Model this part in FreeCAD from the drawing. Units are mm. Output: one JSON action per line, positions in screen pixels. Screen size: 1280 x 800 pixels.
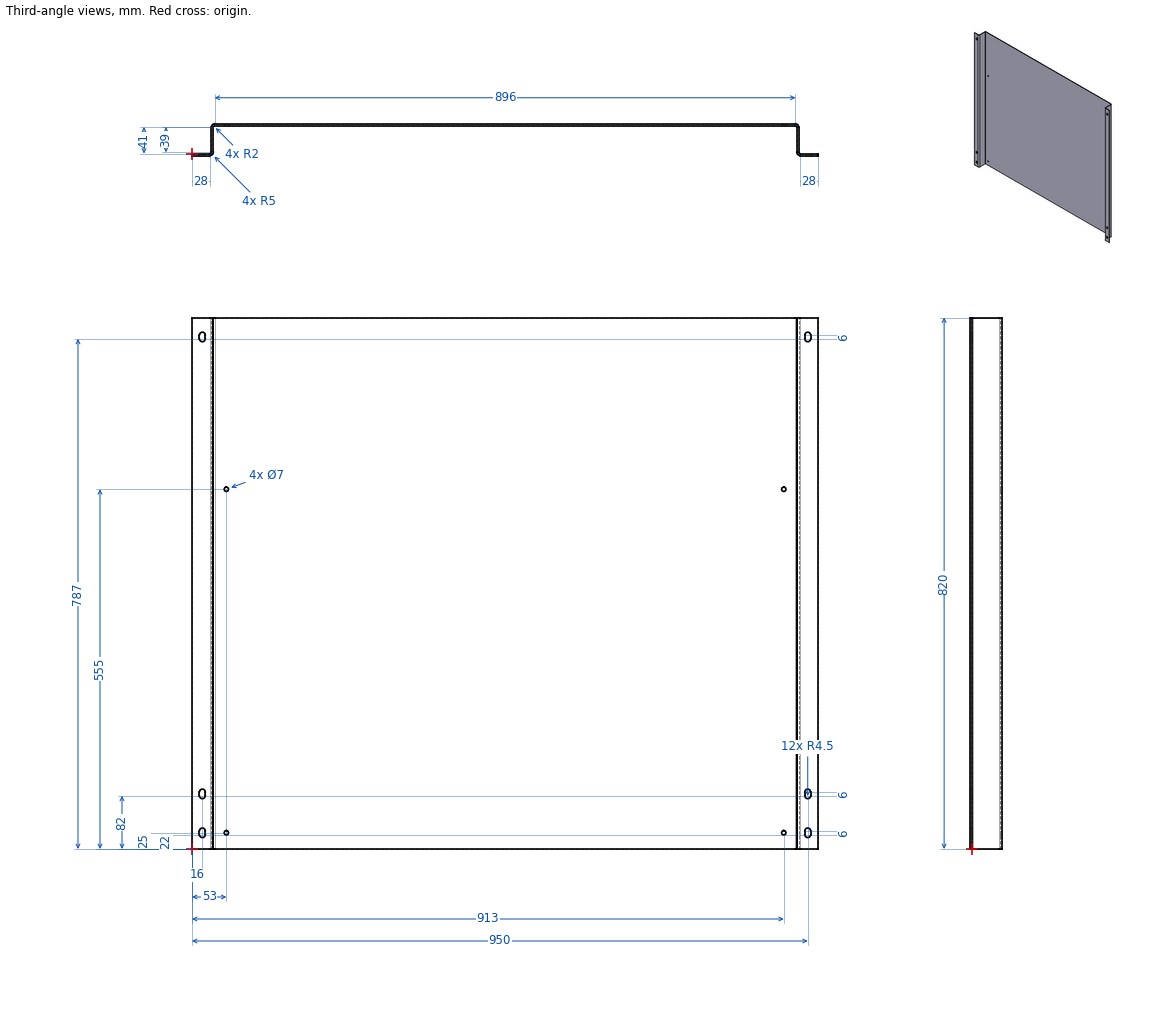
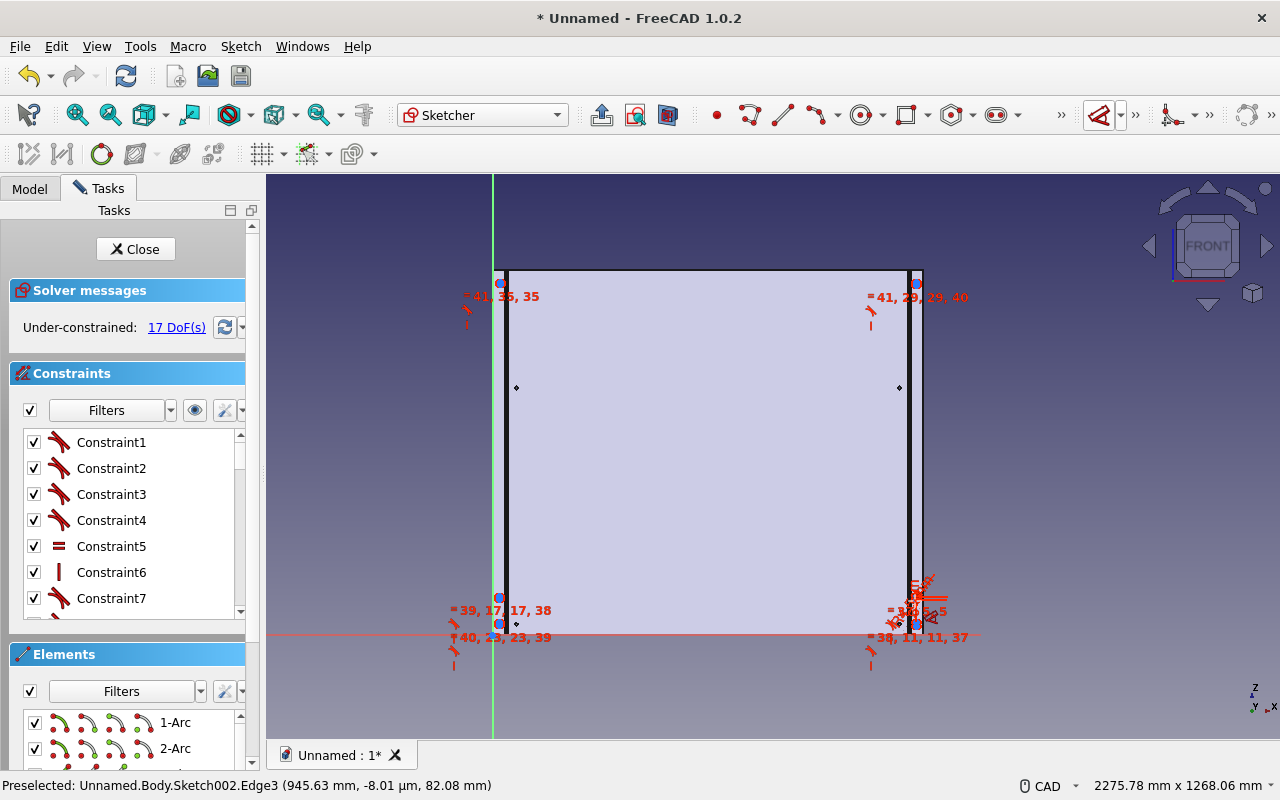
{"action": "scroll", "coordinate": [914, 625], "scroll_direction": "up", "scroll_amount": 14}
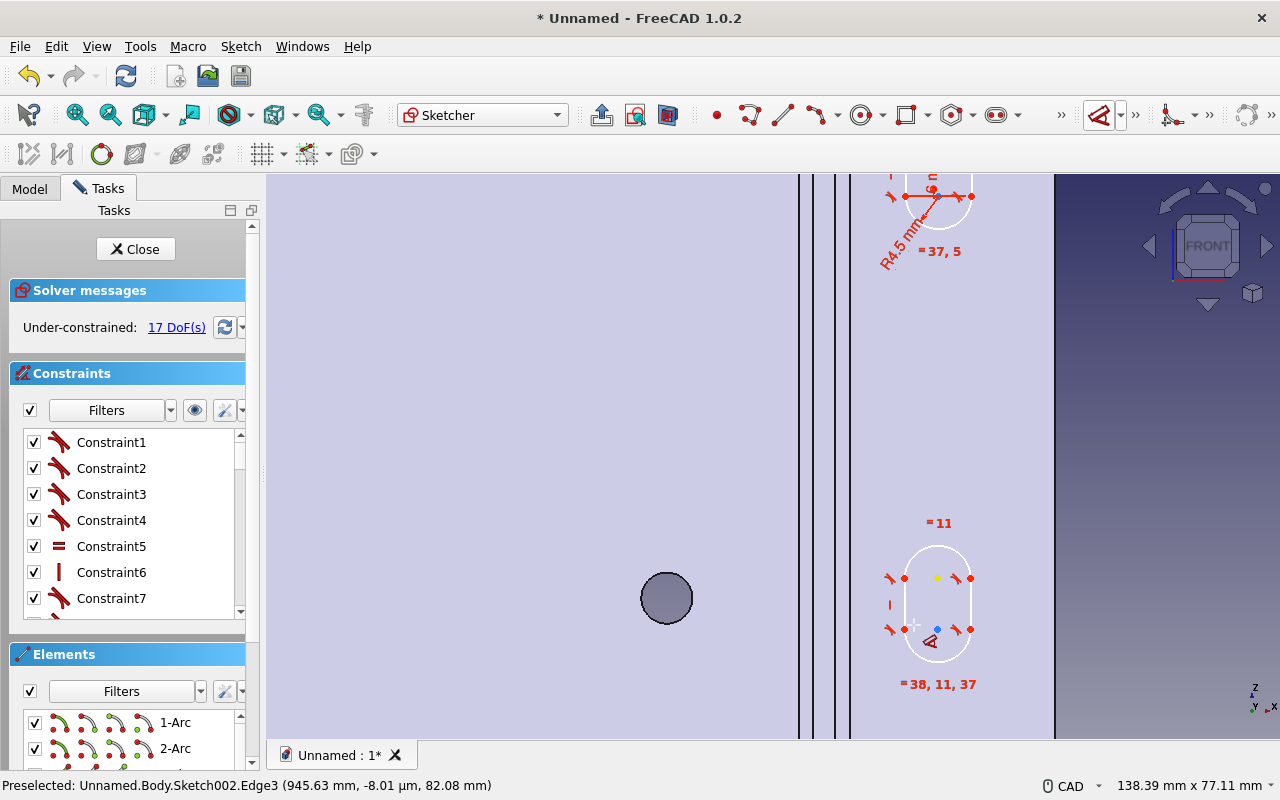
{"action": "left_click", "coordinate": [905, 614]}
{"action": "left_click", "coordinate": [939, 604]}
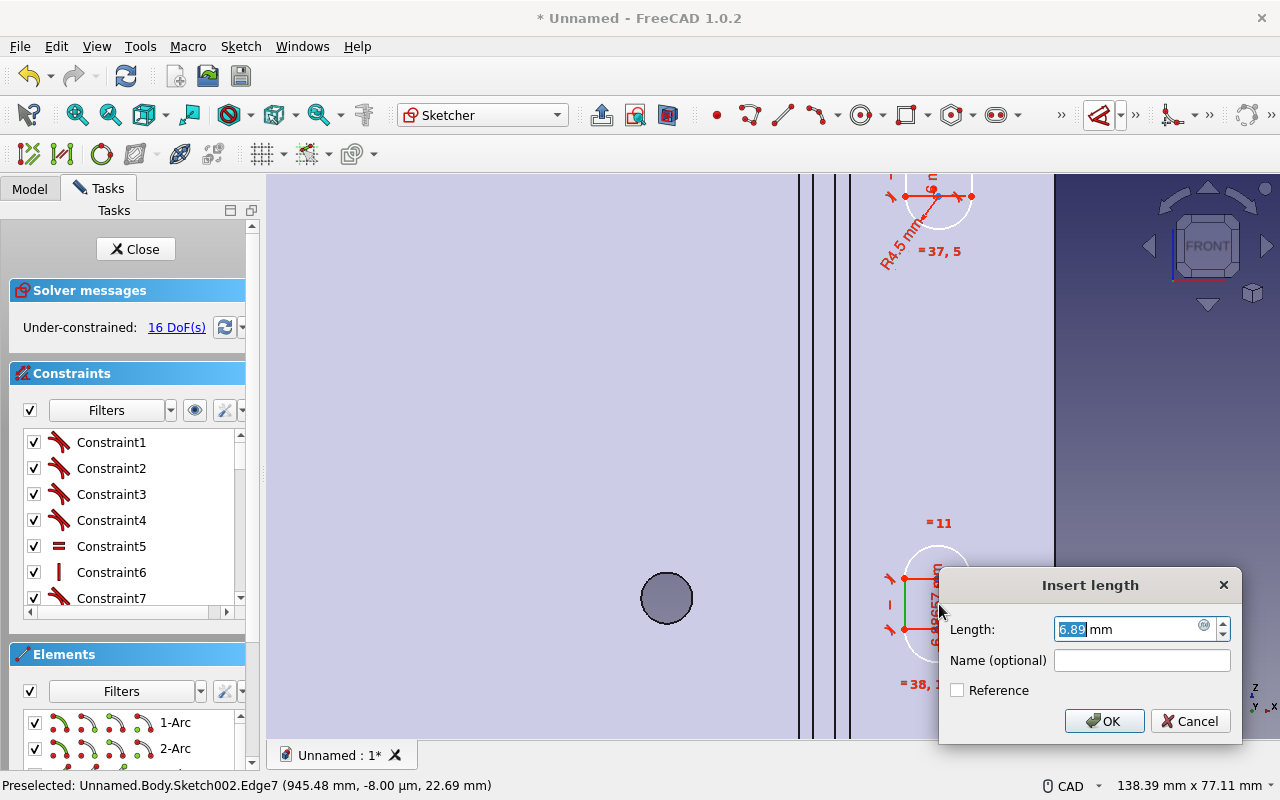
{"action": "type", "text": "6"}
{"action": "key", "text": "Return"}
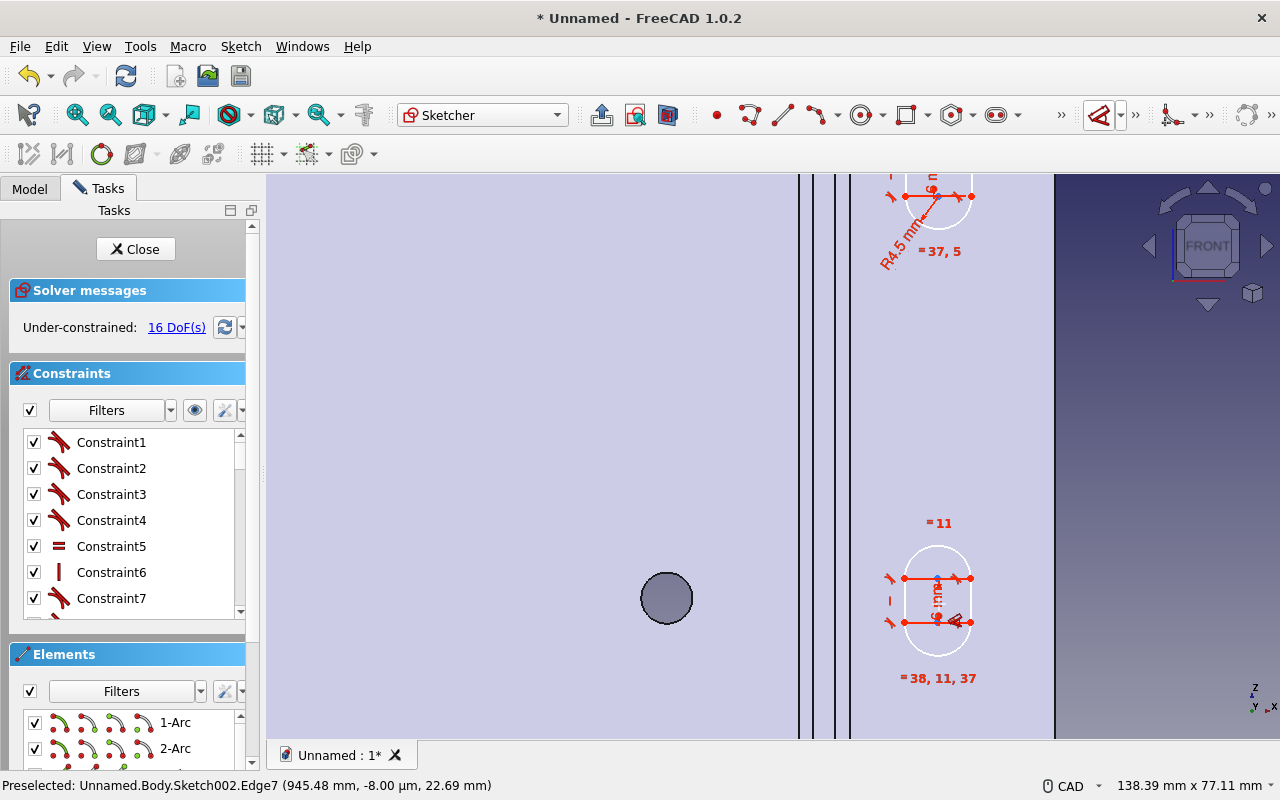
{"action": "scroll", "coordinate": [914, 625], "scroll_direction": "down", "scroll_amount": 14}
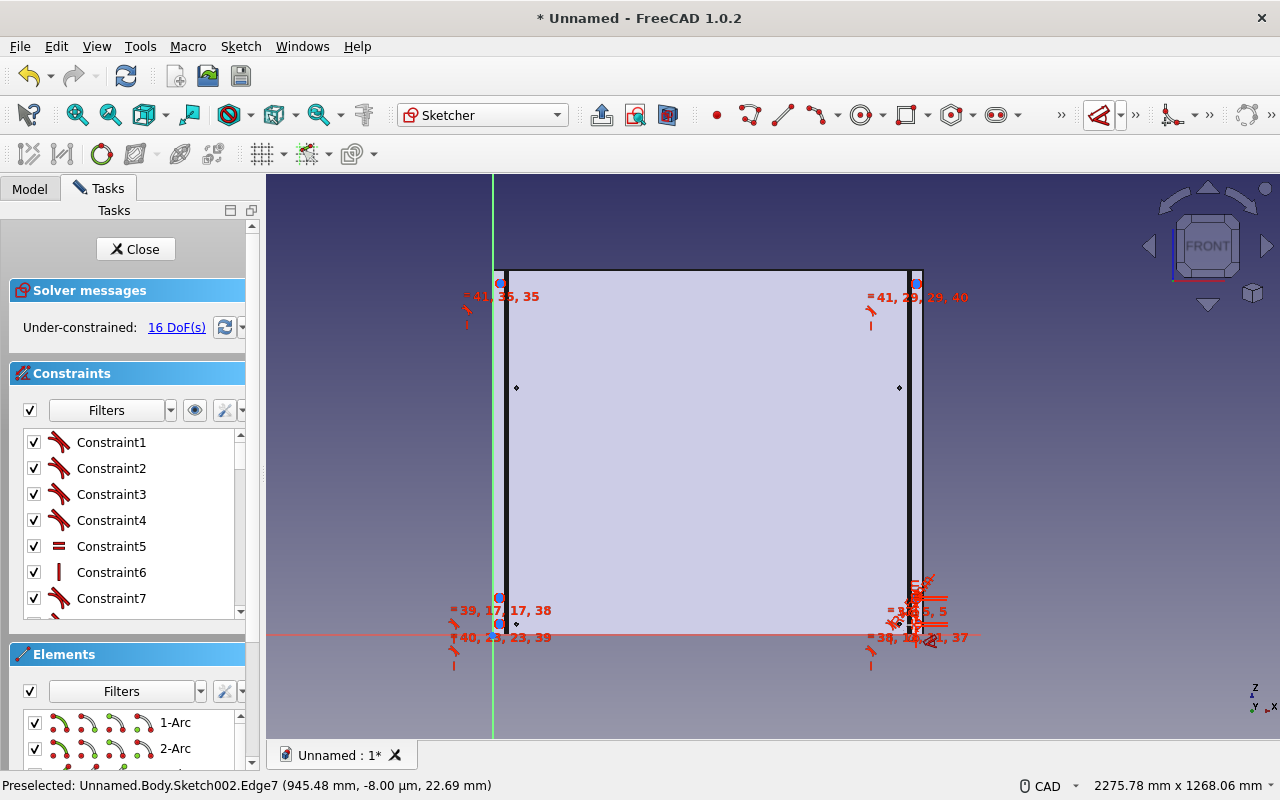
{"action": "scroll", "coordinate": [498, 598], "scroll_direction": "up", "scroll_amount": 14}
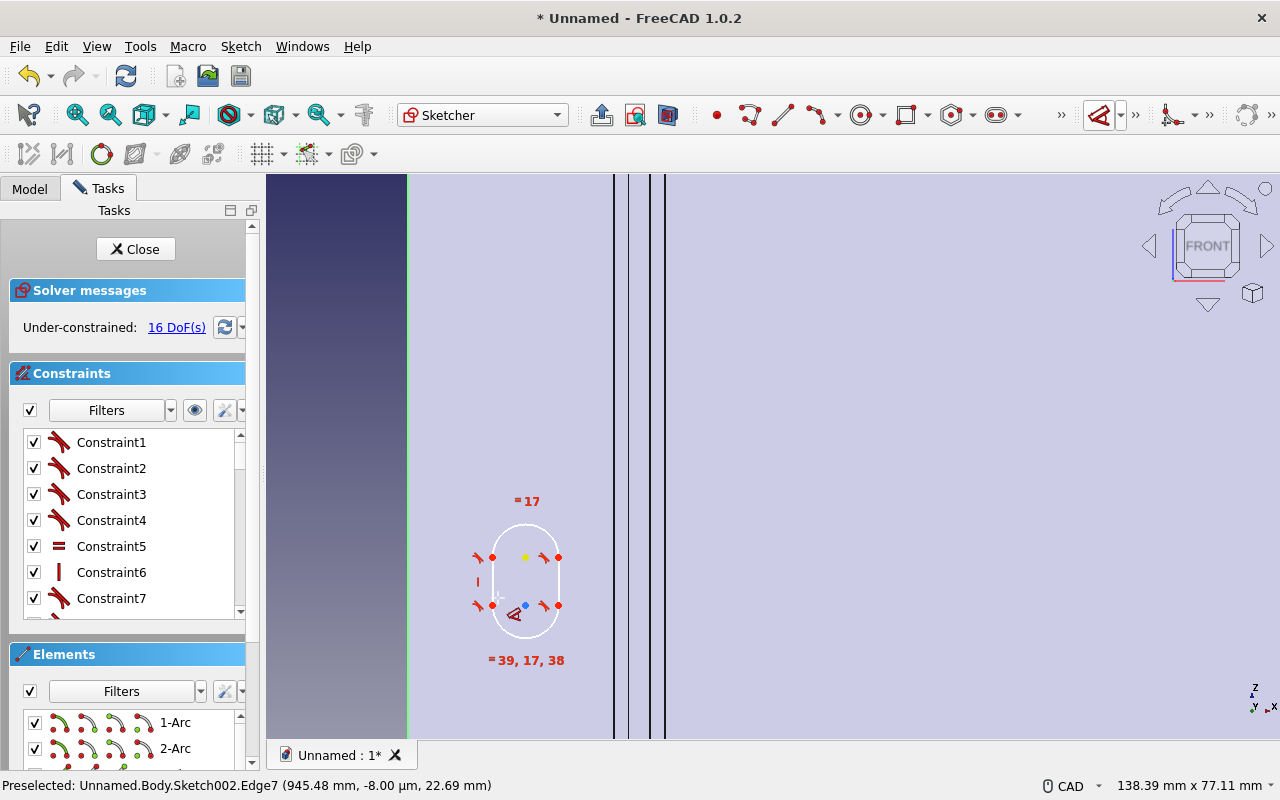
{"action": "left_click", "coordinate": [493, 591]}
{"action": "left_click", "coordinate": [459, 581]}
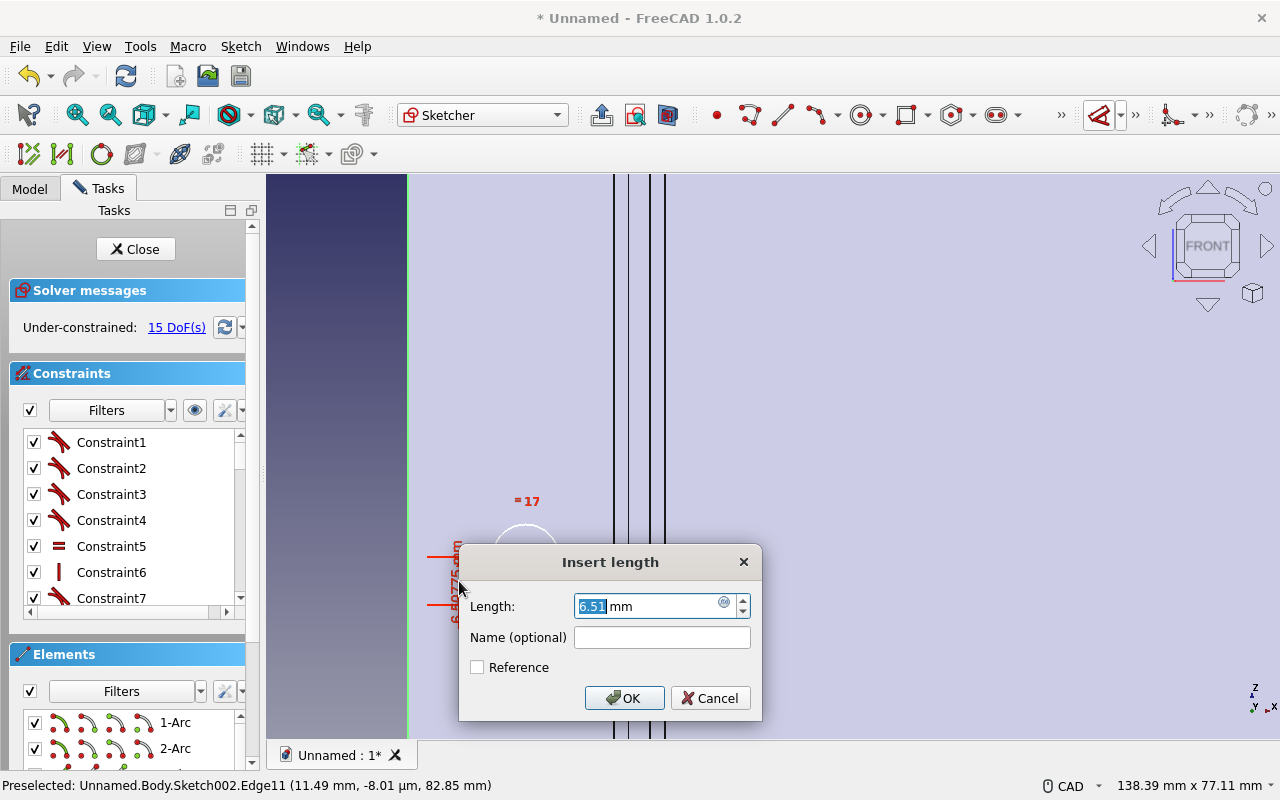
{"action": "type", "text": "6"}
{"action": "key", "text": "Return"}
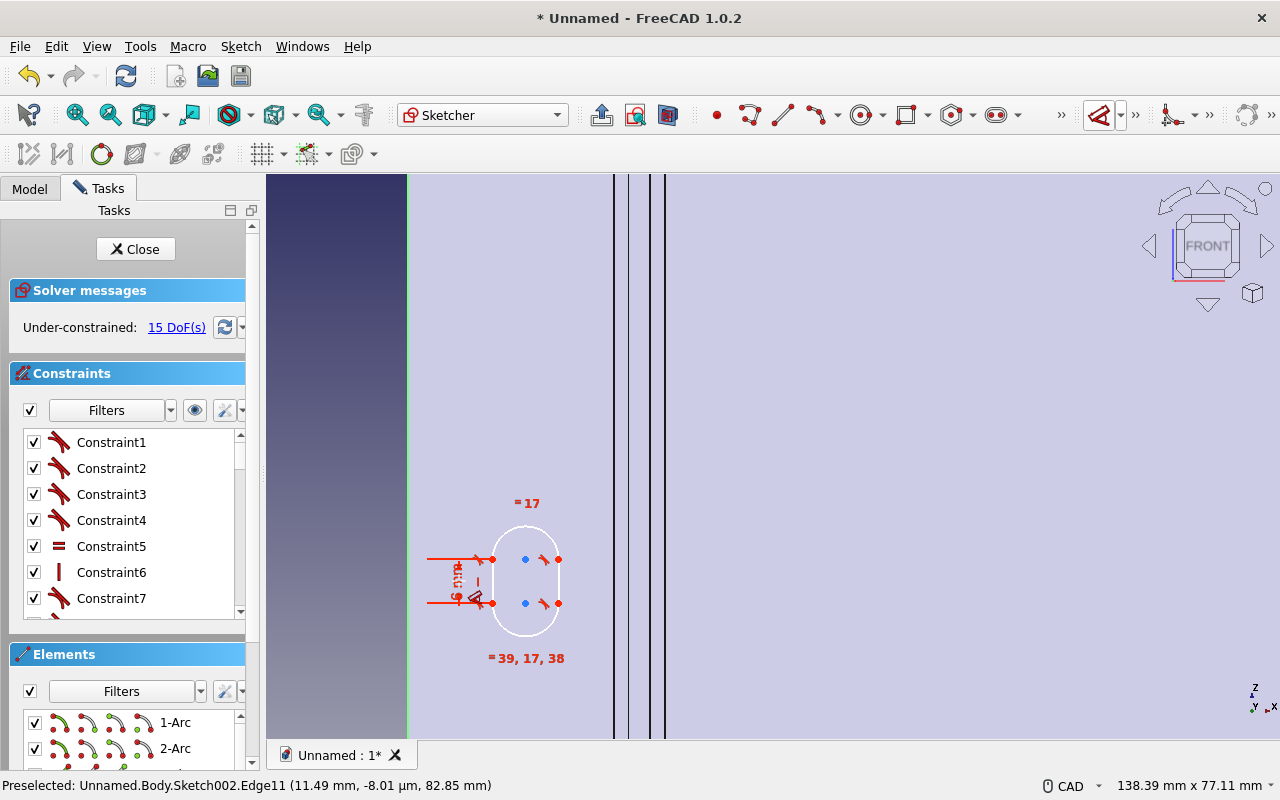
{"action": "scroll", "coordinate": [497, 598], "scroll_direction": "down", "scroll_amount": 14}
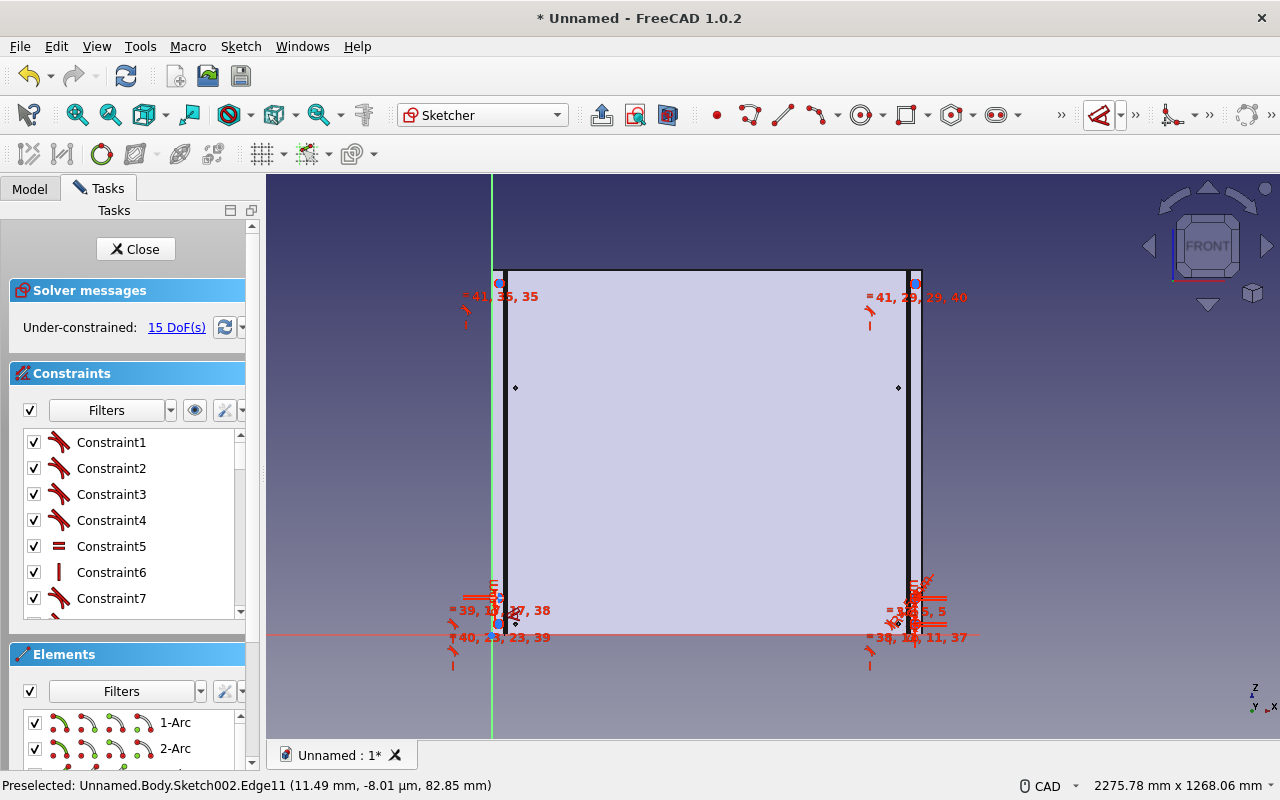
{"action": "scroll", "coordinate": [497, 625], "scroll_direction": "up", "scroll_amount": 14}